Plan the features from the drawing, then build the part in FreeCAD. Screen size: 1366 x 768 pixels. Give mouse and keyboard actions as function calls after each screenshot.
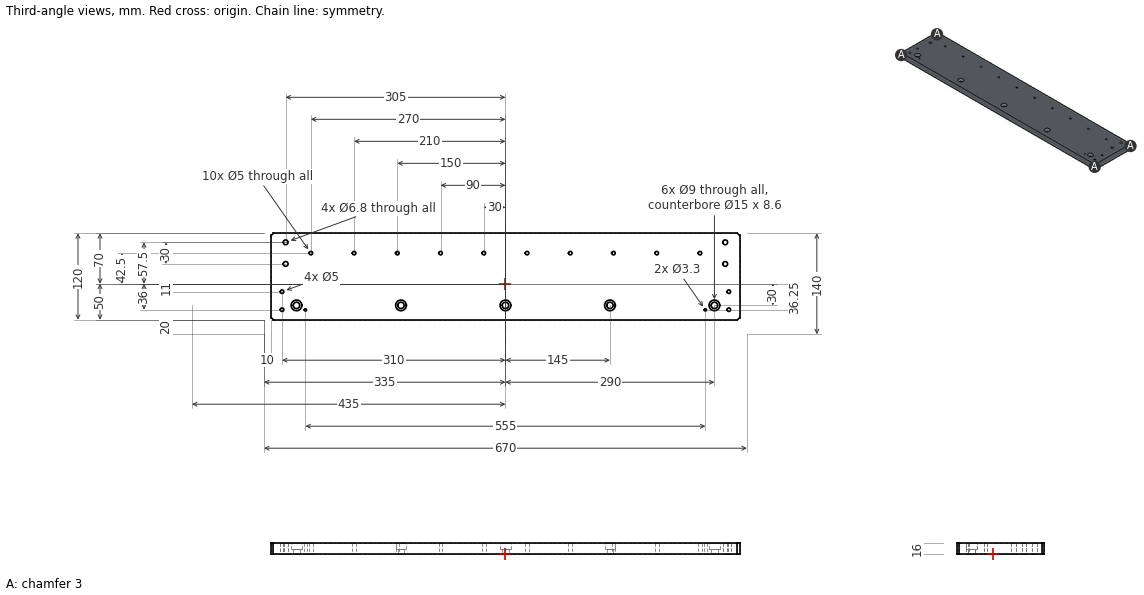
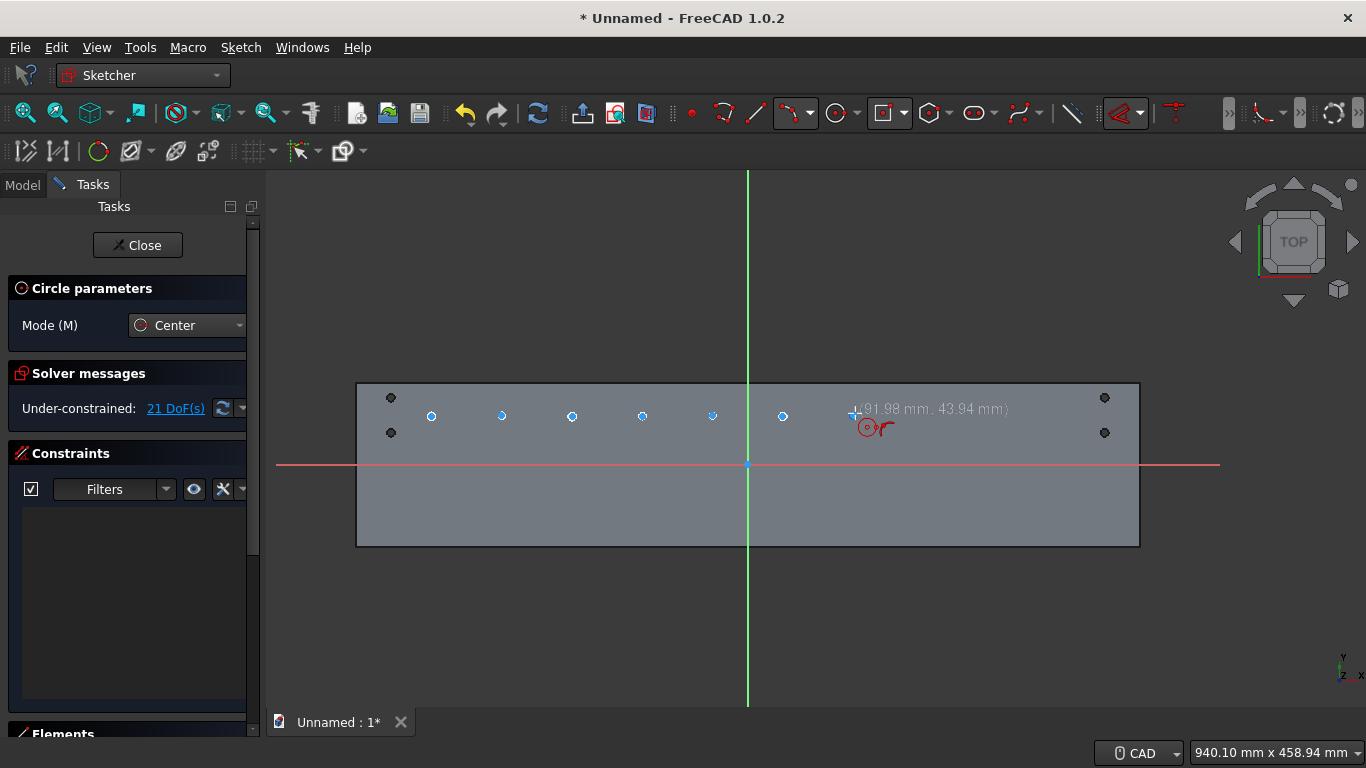
scroll(923, 415, up, 11)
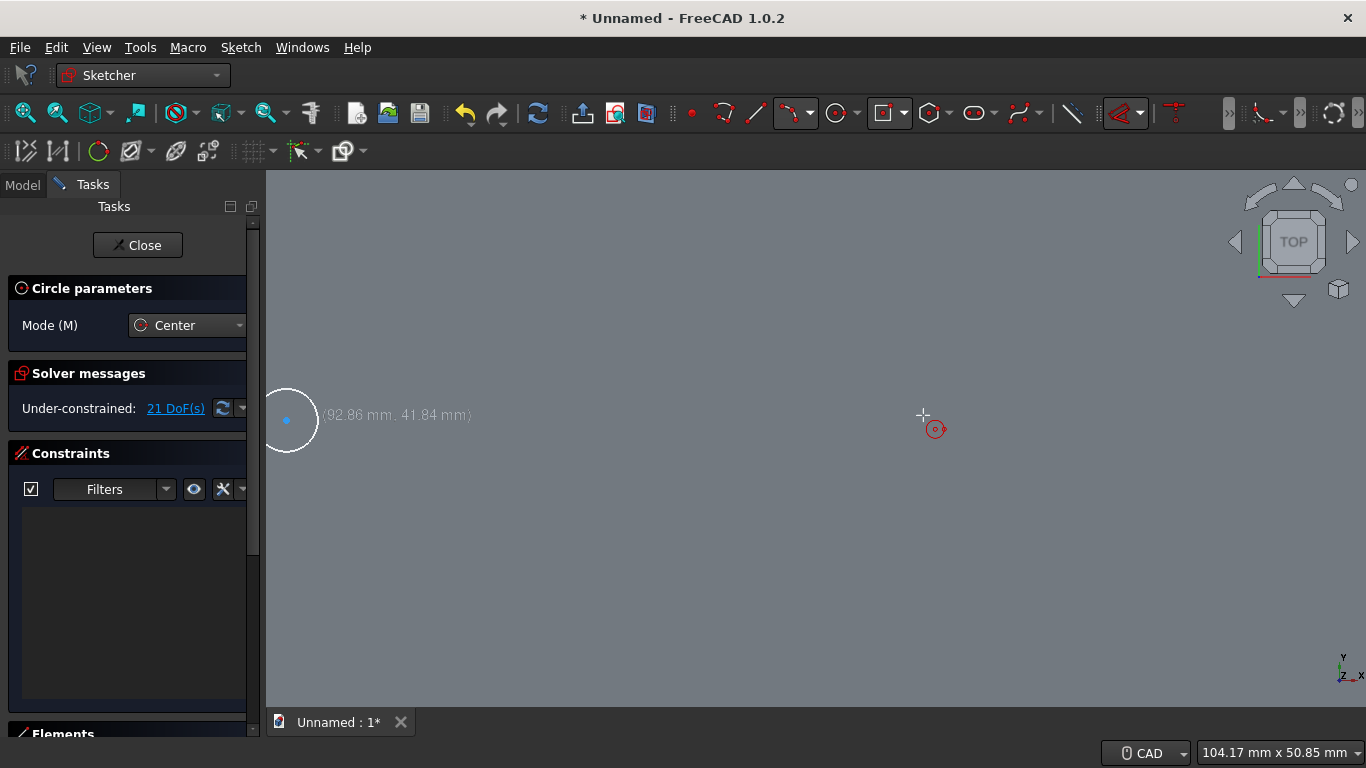
scroll(923, 415, down, 11)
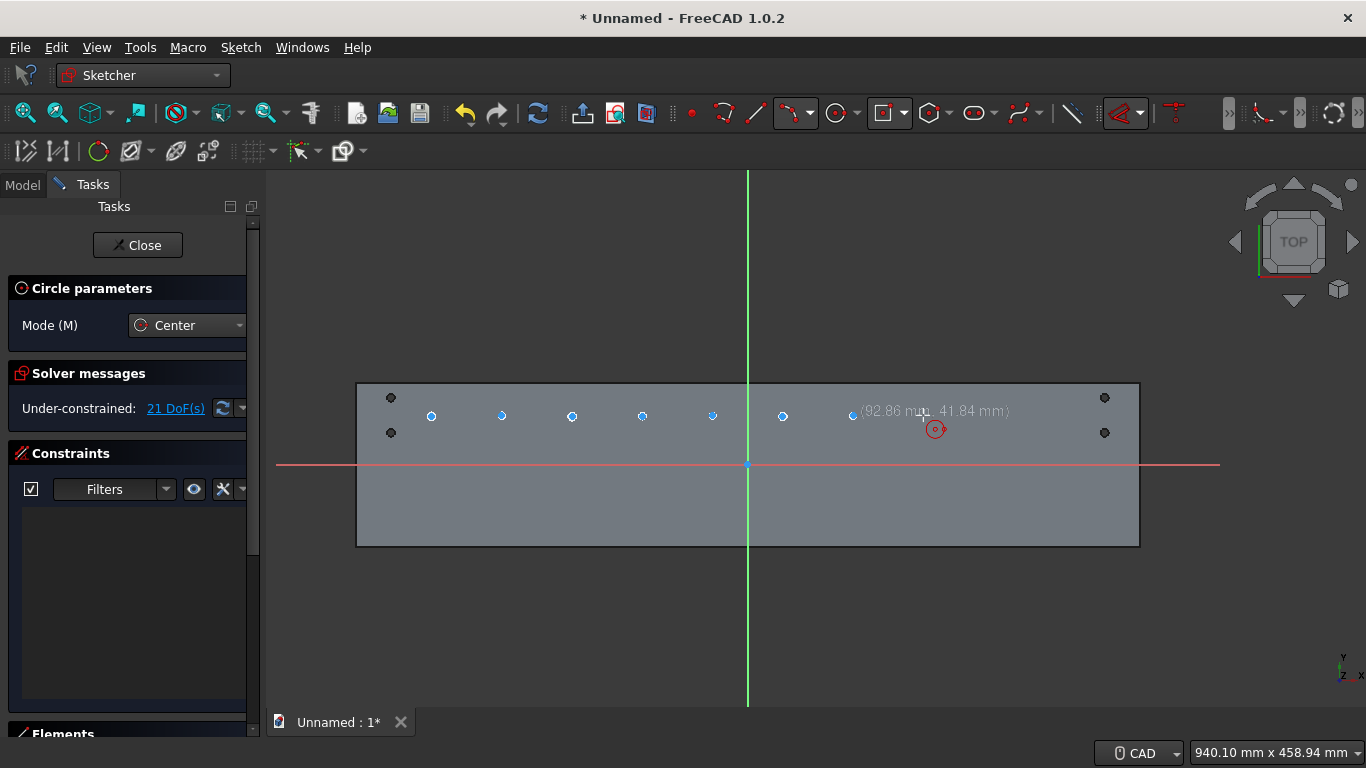
click(923, 415)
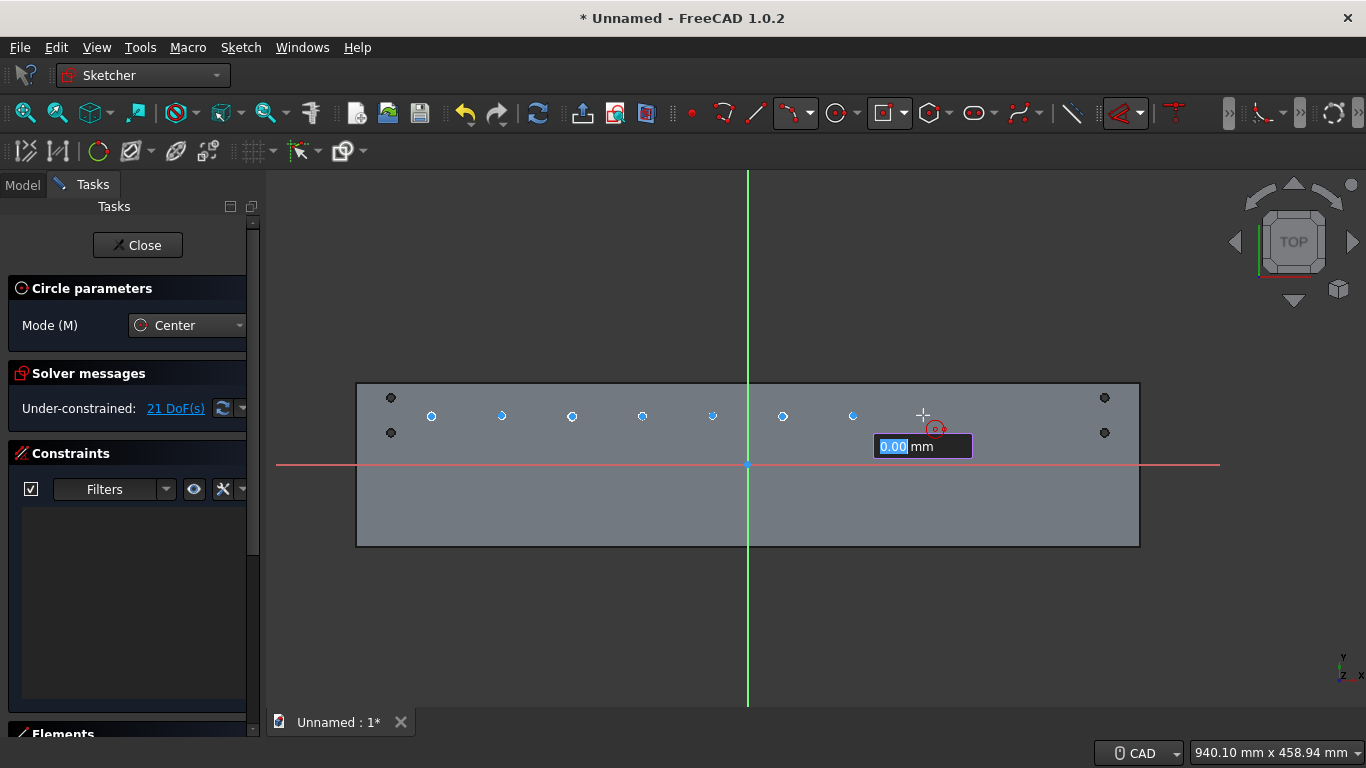
scroll(925, 413, up, 9)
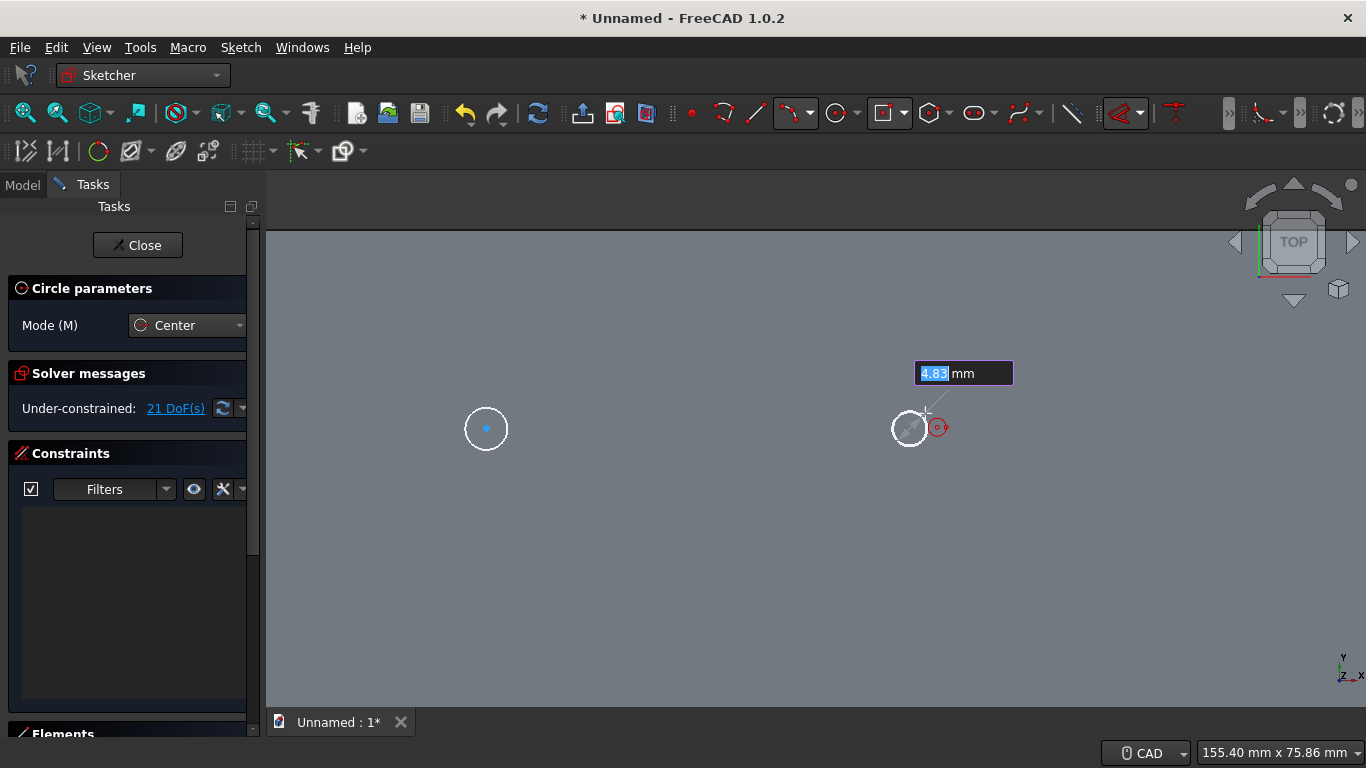
click(924, 412)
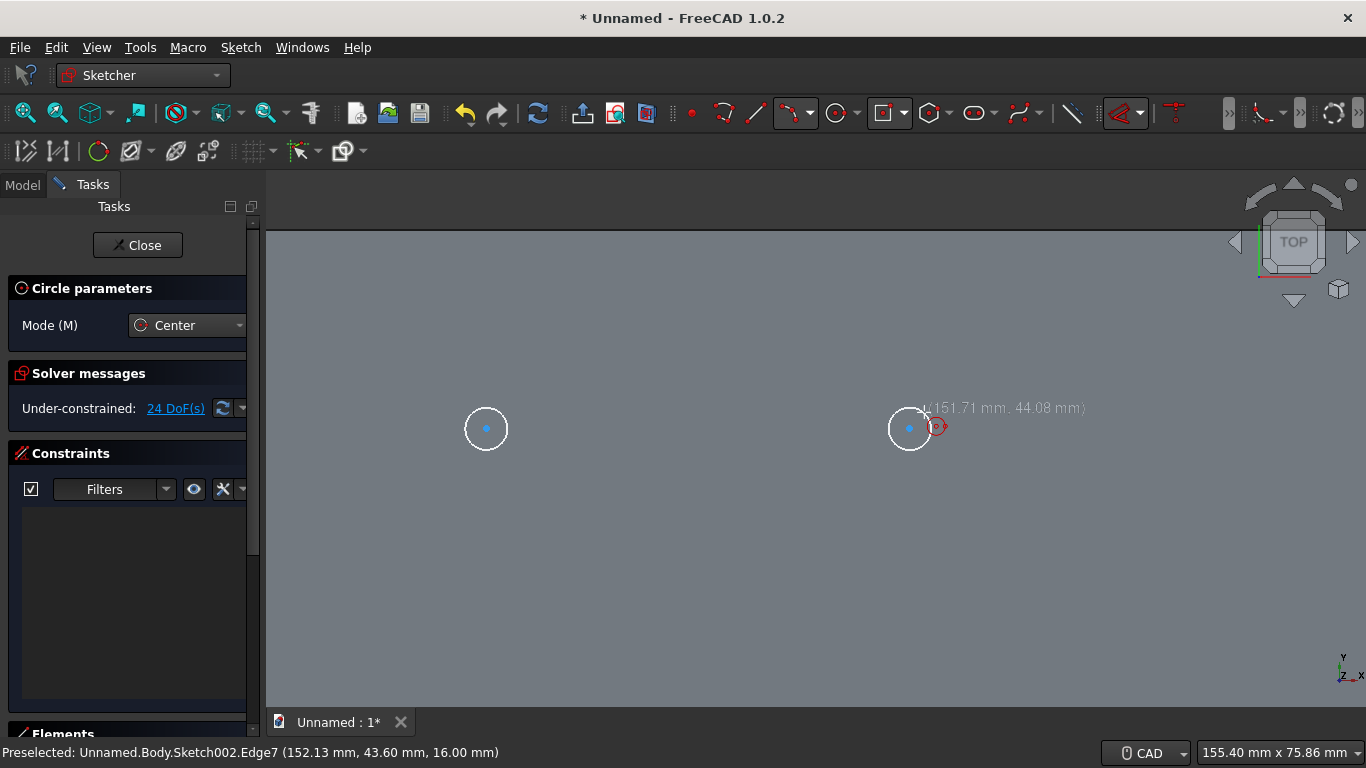
scroll(925, 413, down, 9)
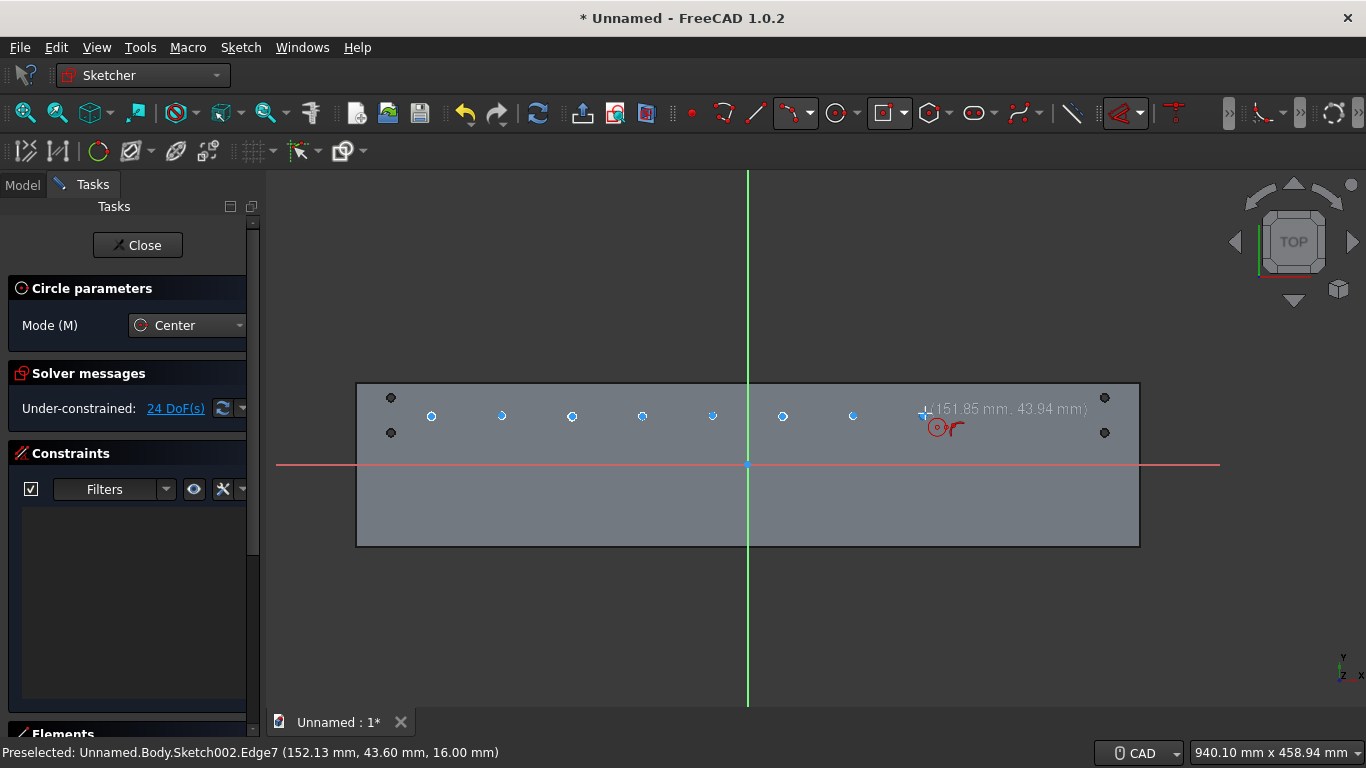
scroll(994, 415, up, 11)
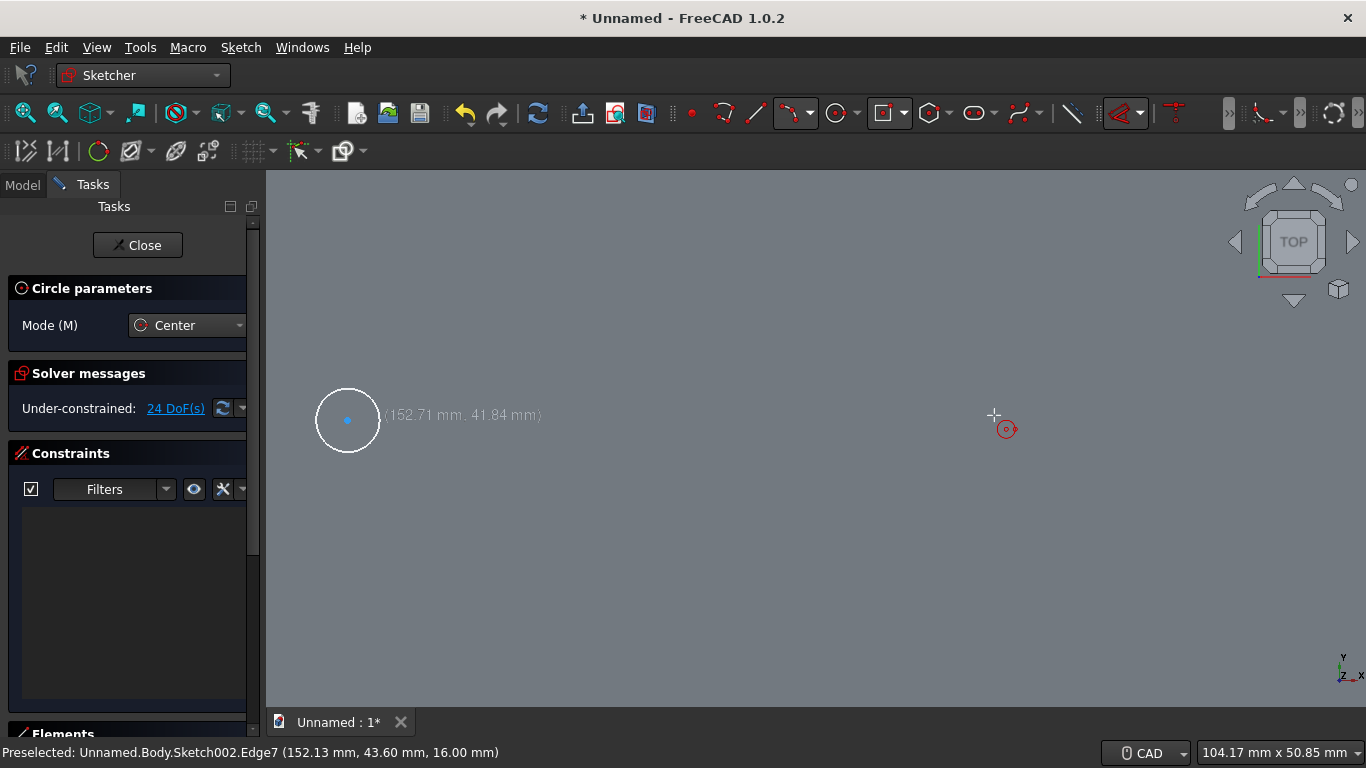
scroll(994, 415, down, 11)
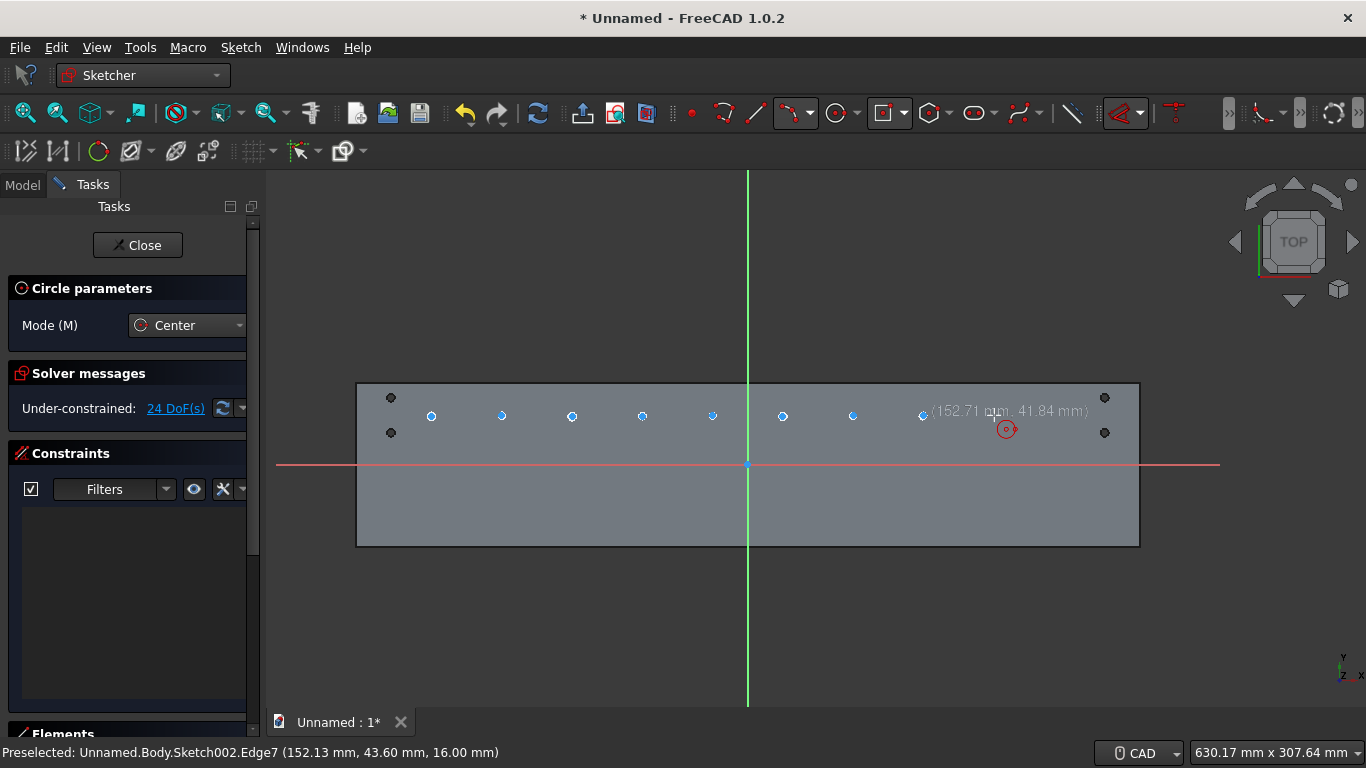
click(994, 415)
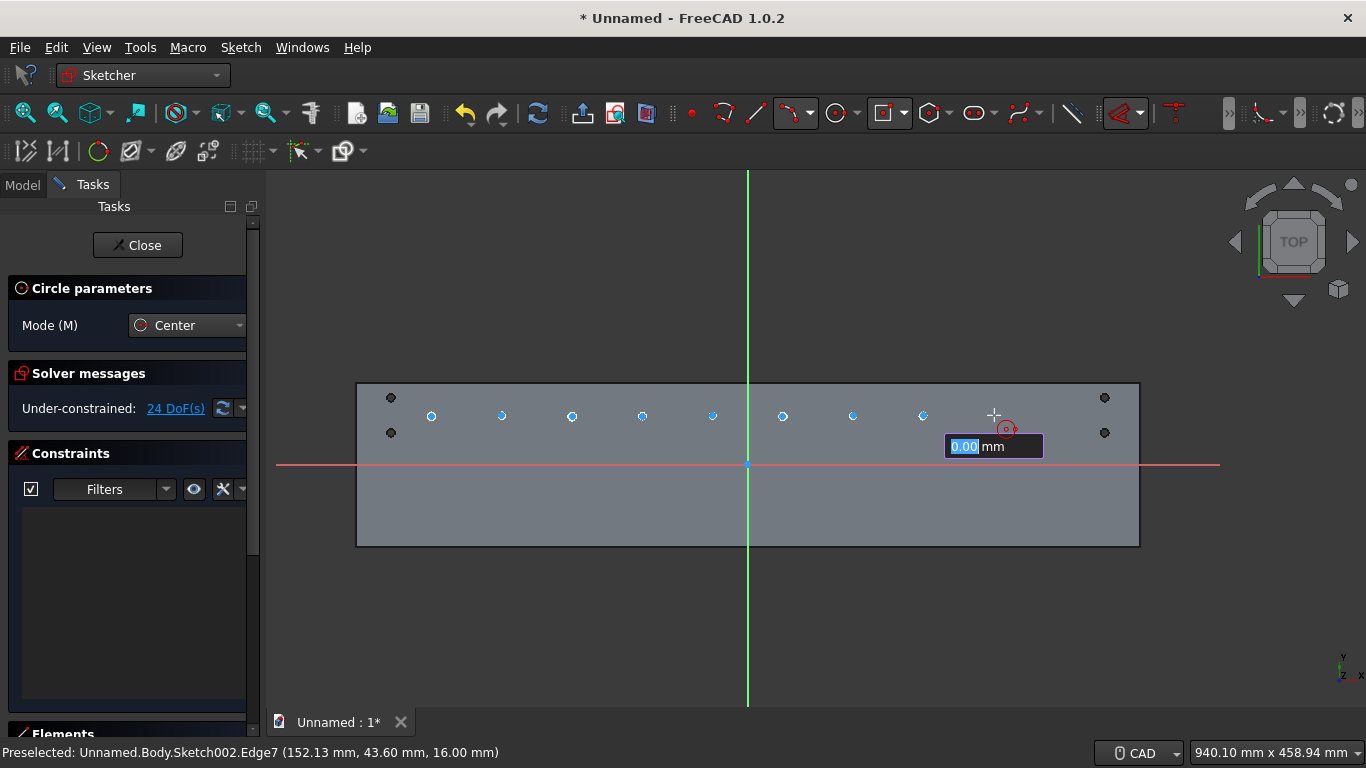
scroll(996, 413, up, 9)